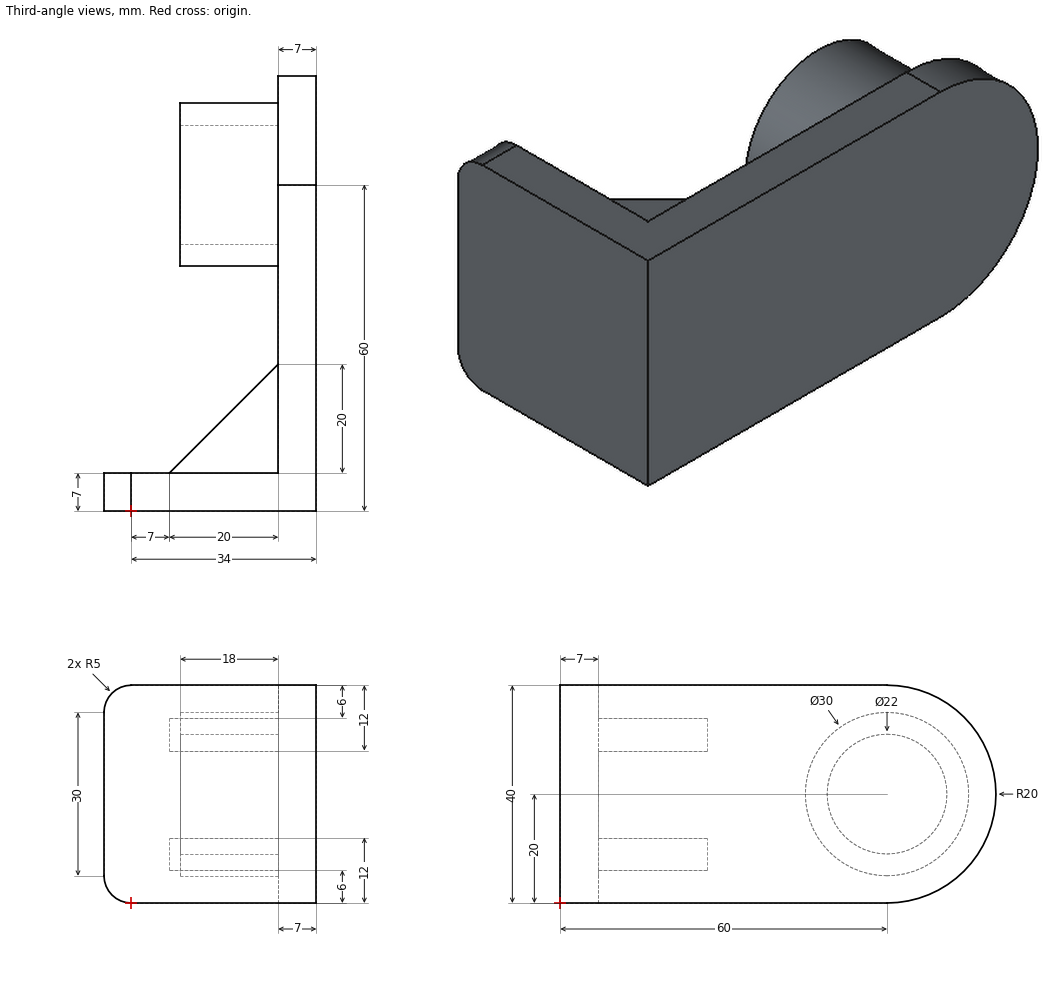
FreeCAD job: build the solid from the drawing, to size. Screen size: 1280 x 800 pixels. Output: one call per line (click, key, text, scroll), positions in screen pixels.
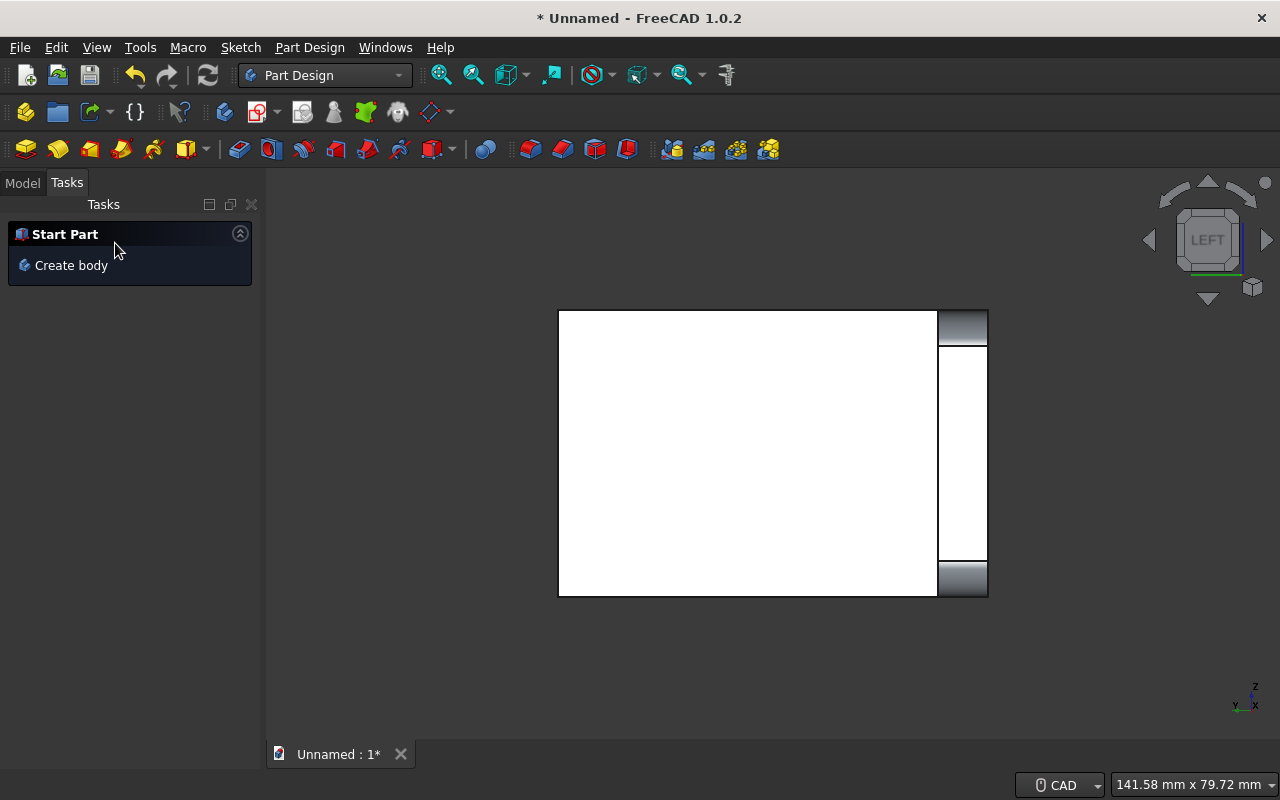
click(748, 453)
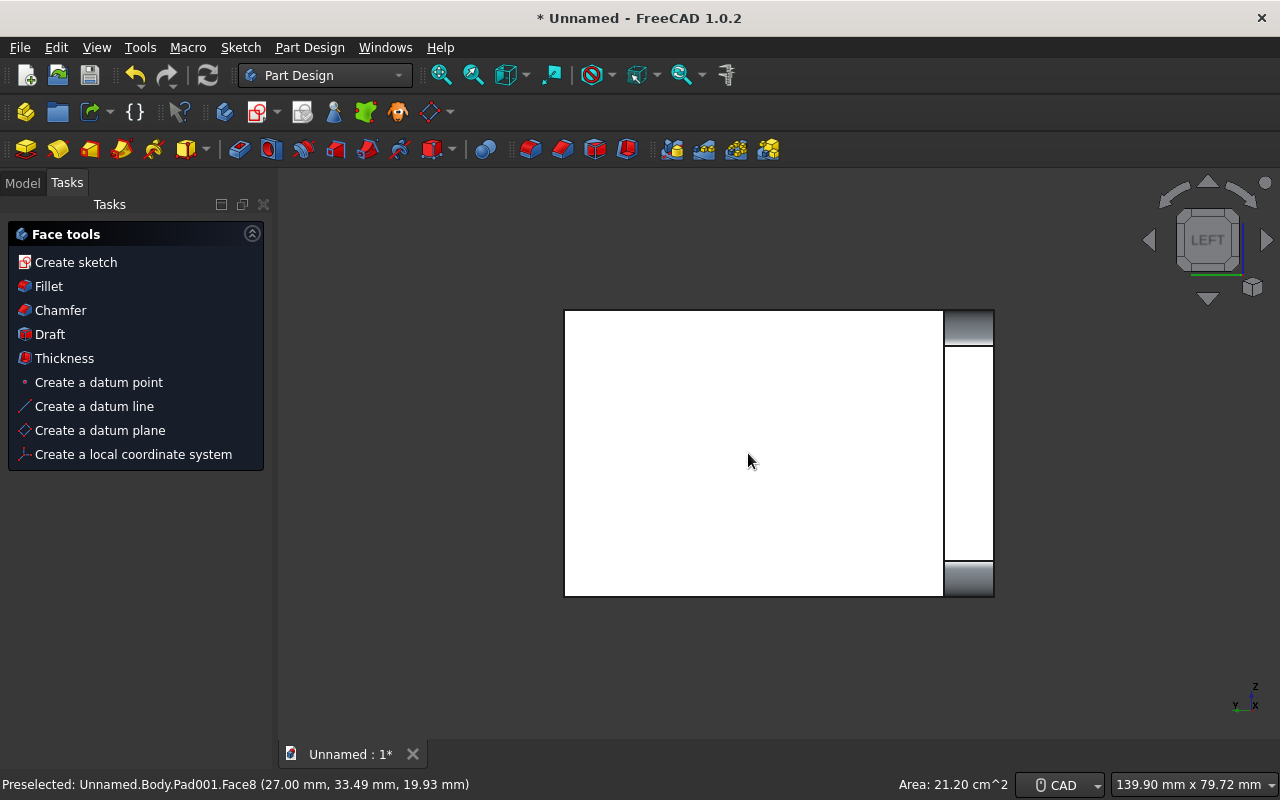
click(258, 112)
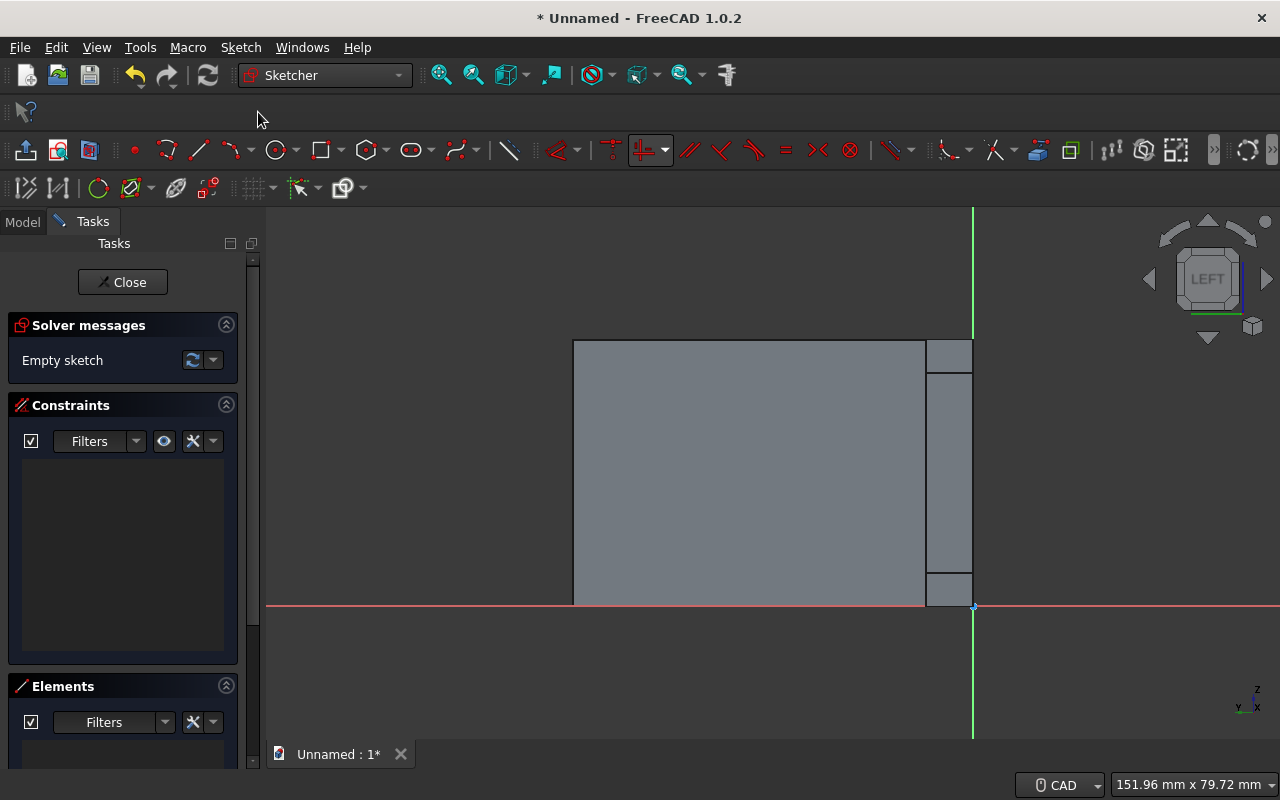
click(90, 150)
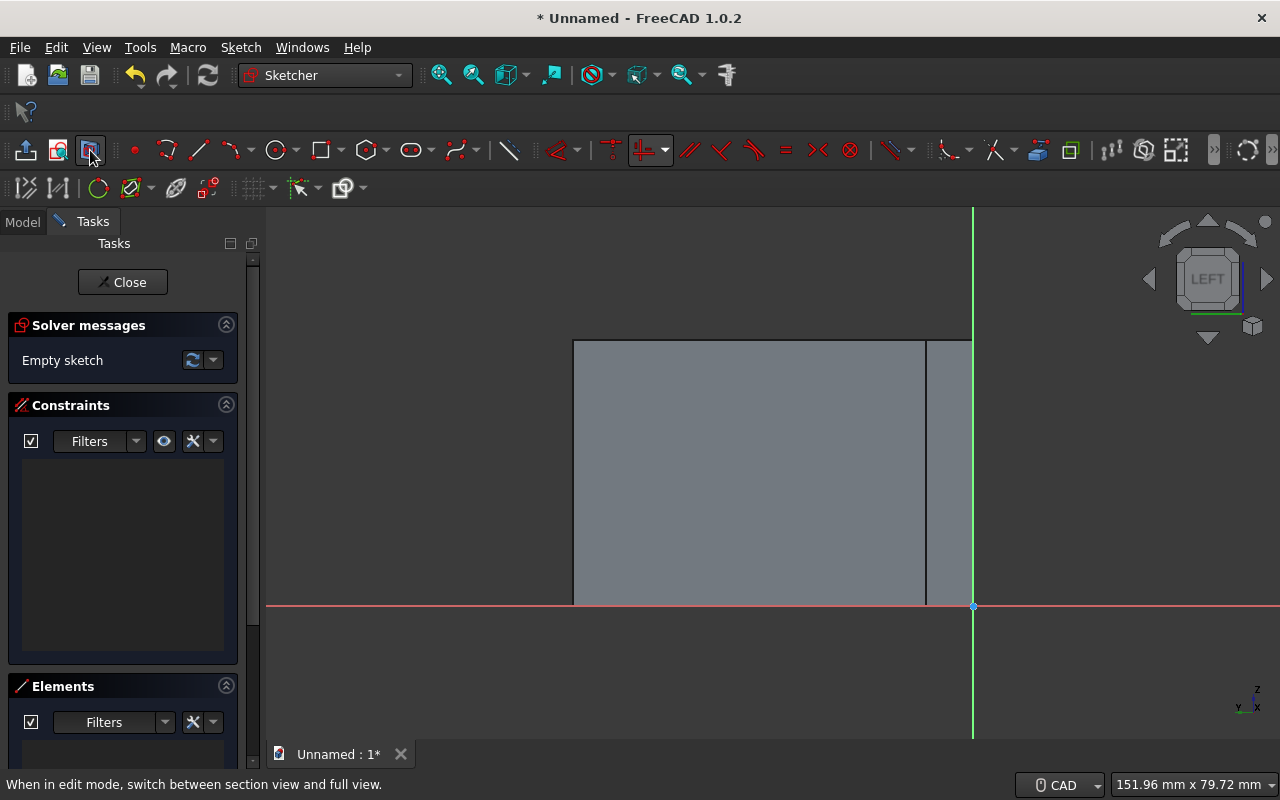
click(200, 150)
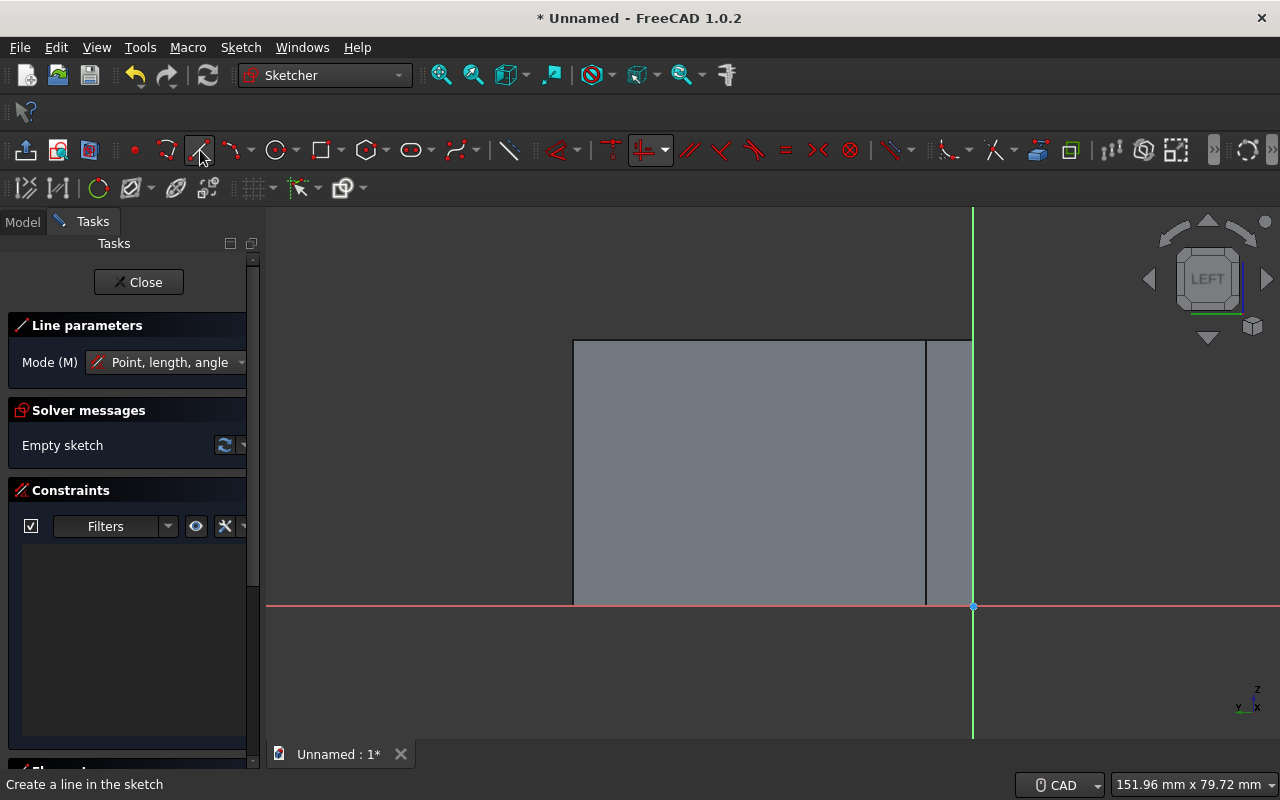
click(573, 606)
click(573, 340)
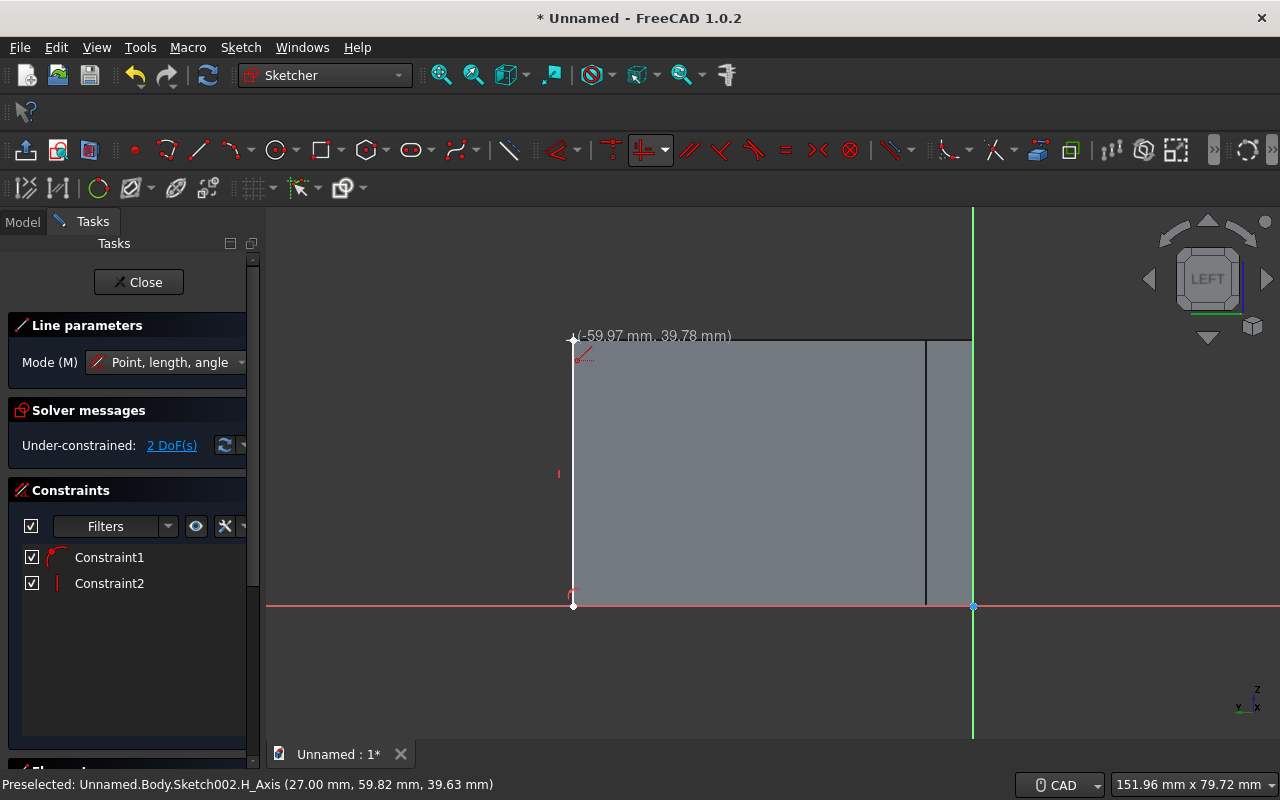
click(232, 150)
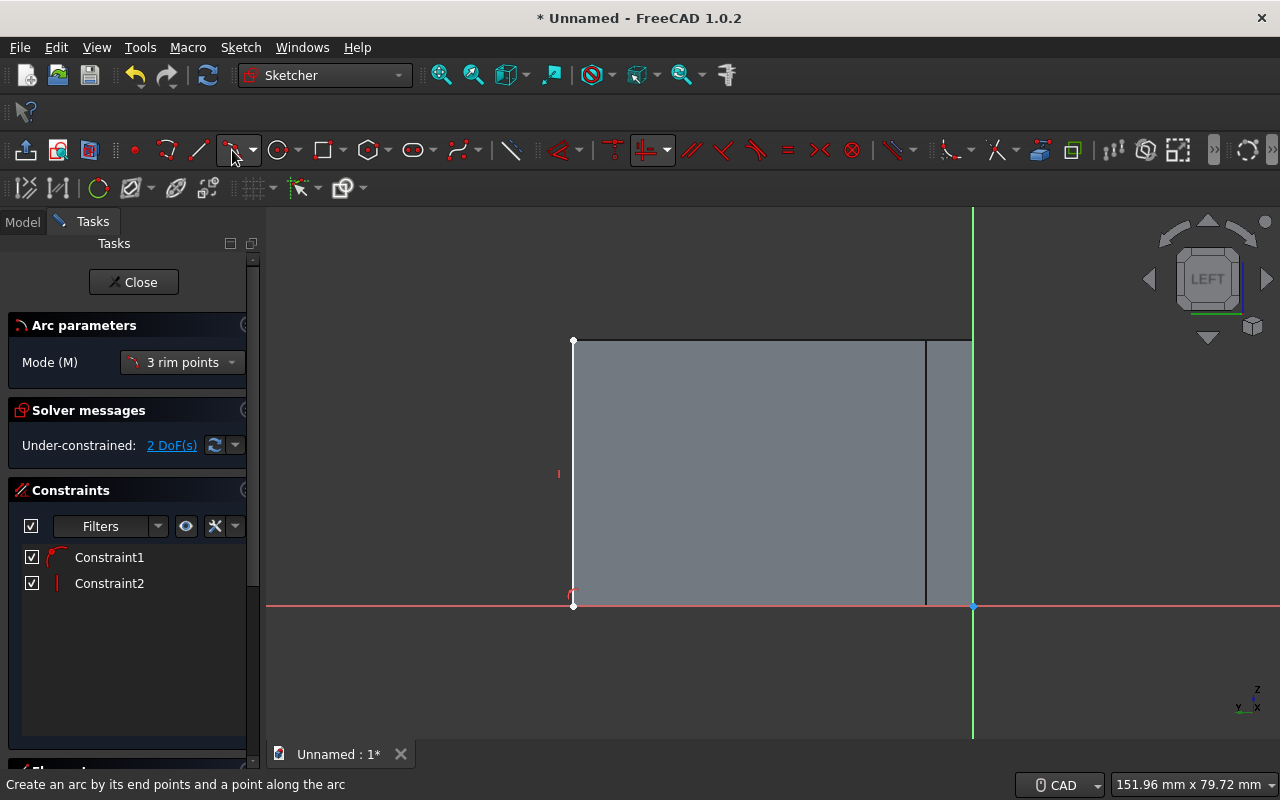
click(573, 341)
click(573, 606)
click(439, 473)
key(Escape)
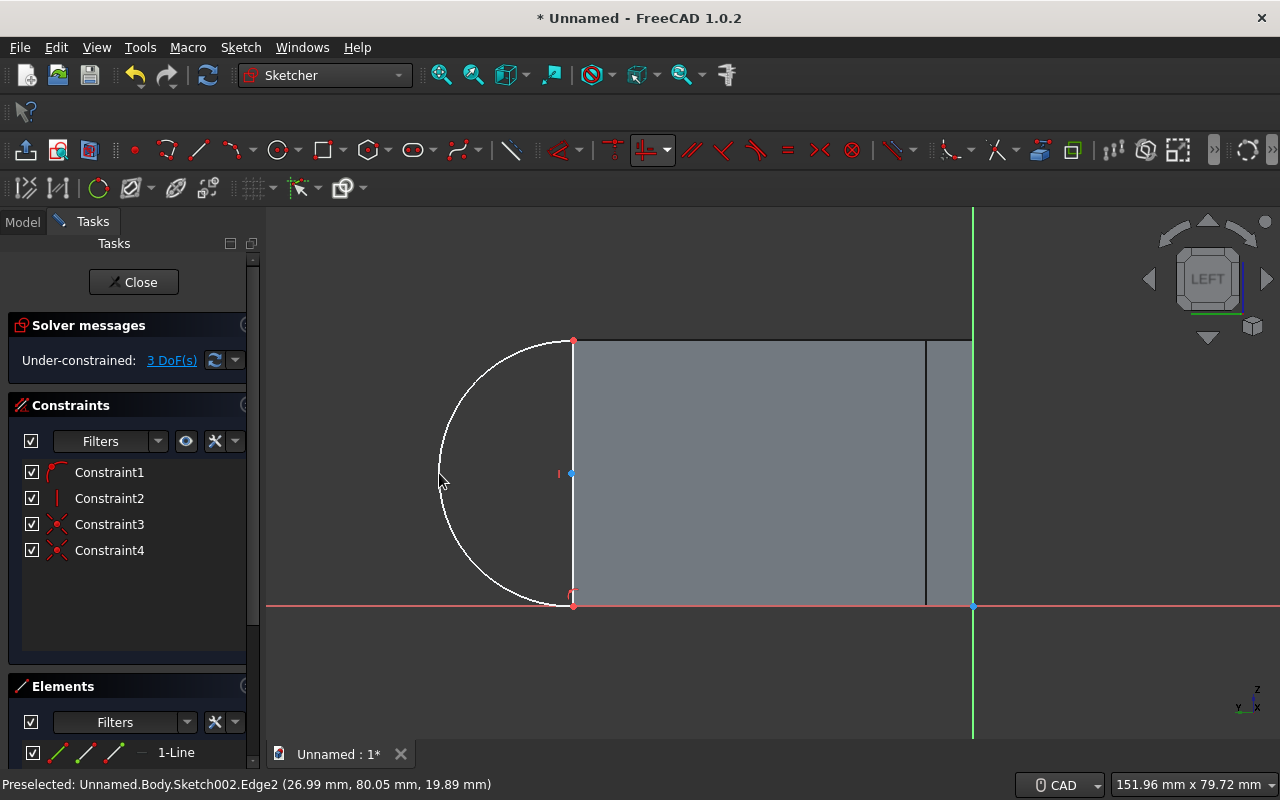
click(558, 150)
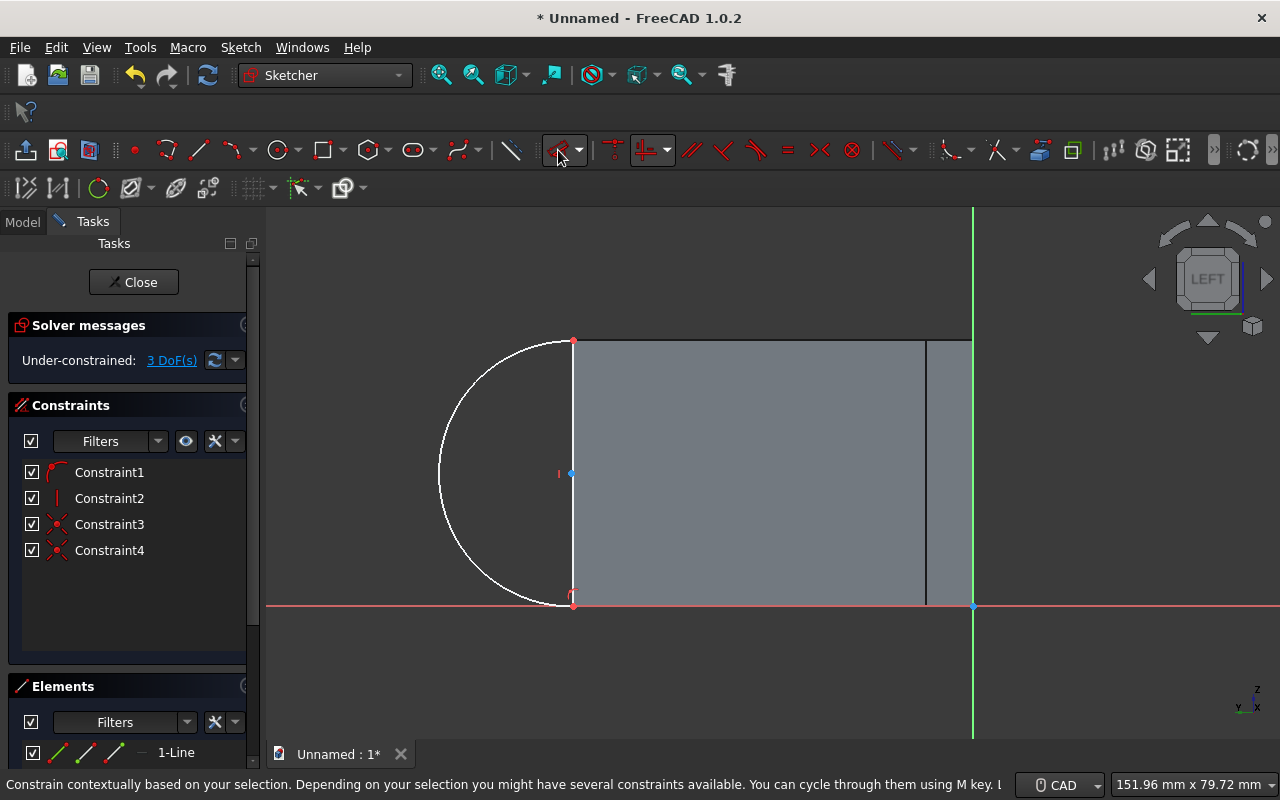
click(465, 395)
click(439, 376)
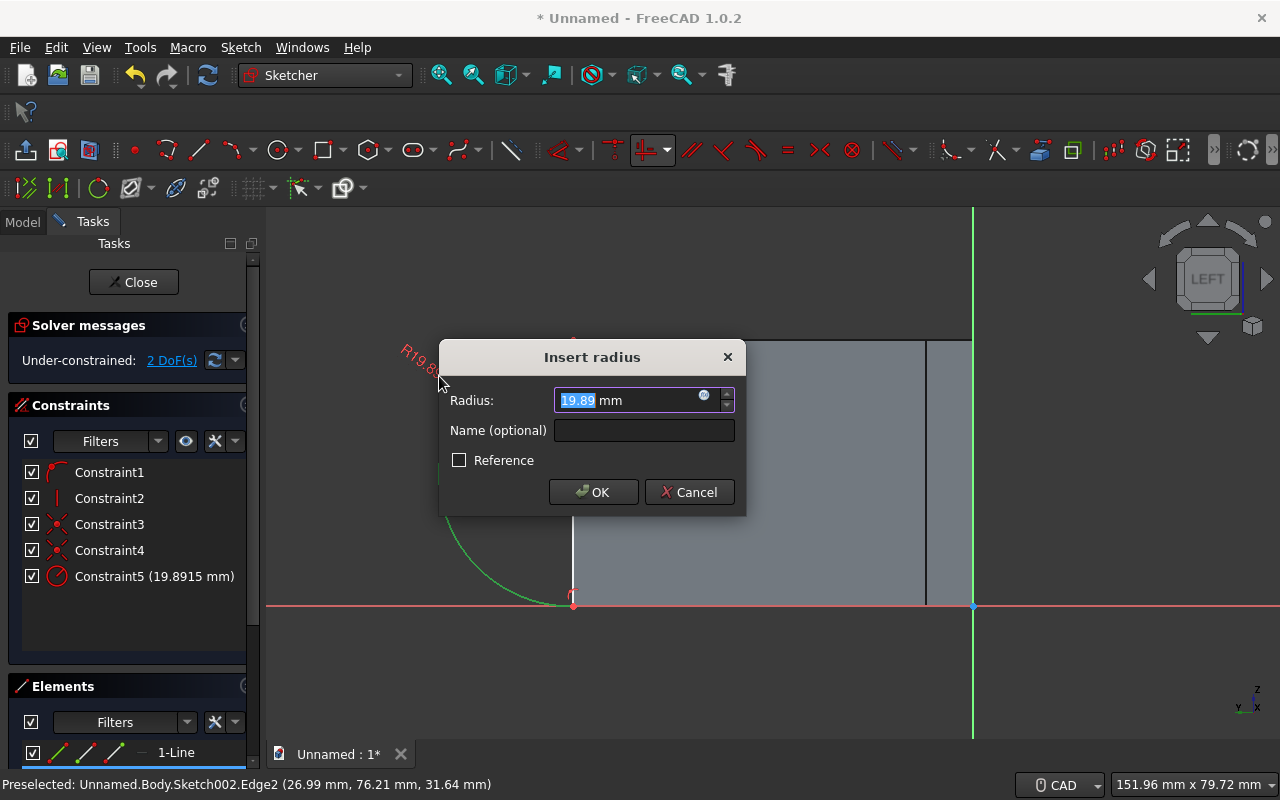
text(20)
key(Return)